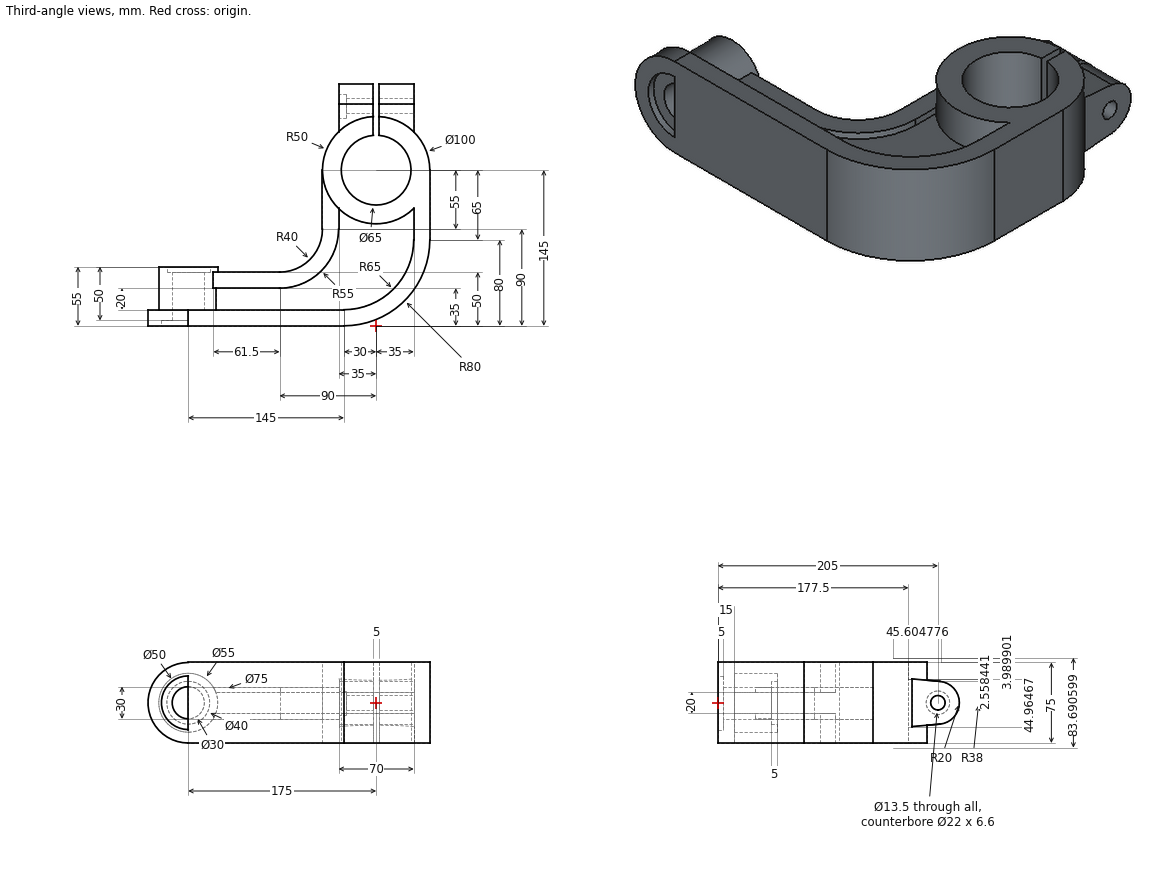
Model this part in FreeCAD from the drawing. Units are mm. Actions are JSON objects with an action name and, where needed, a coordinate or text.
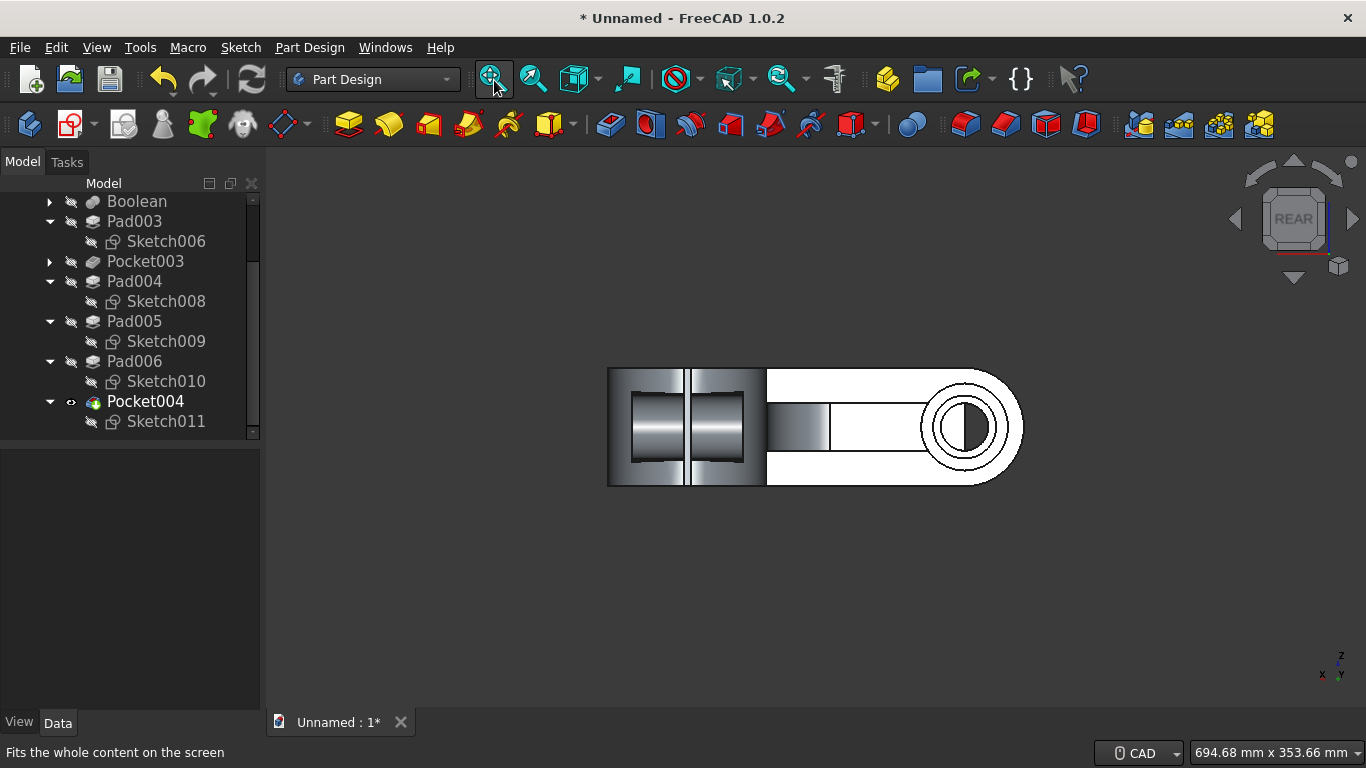
{"action": "key", "text": "6"}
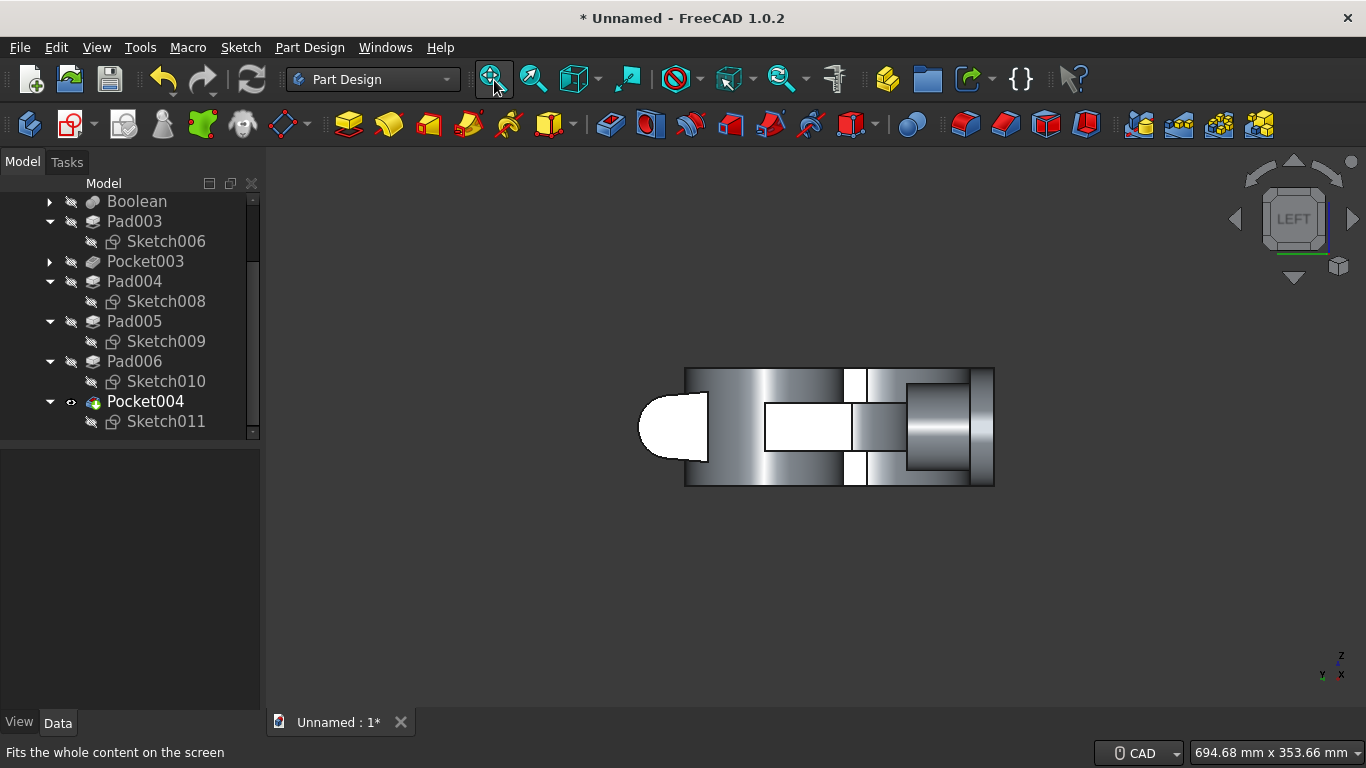
{"action": "key", "text": "v f"}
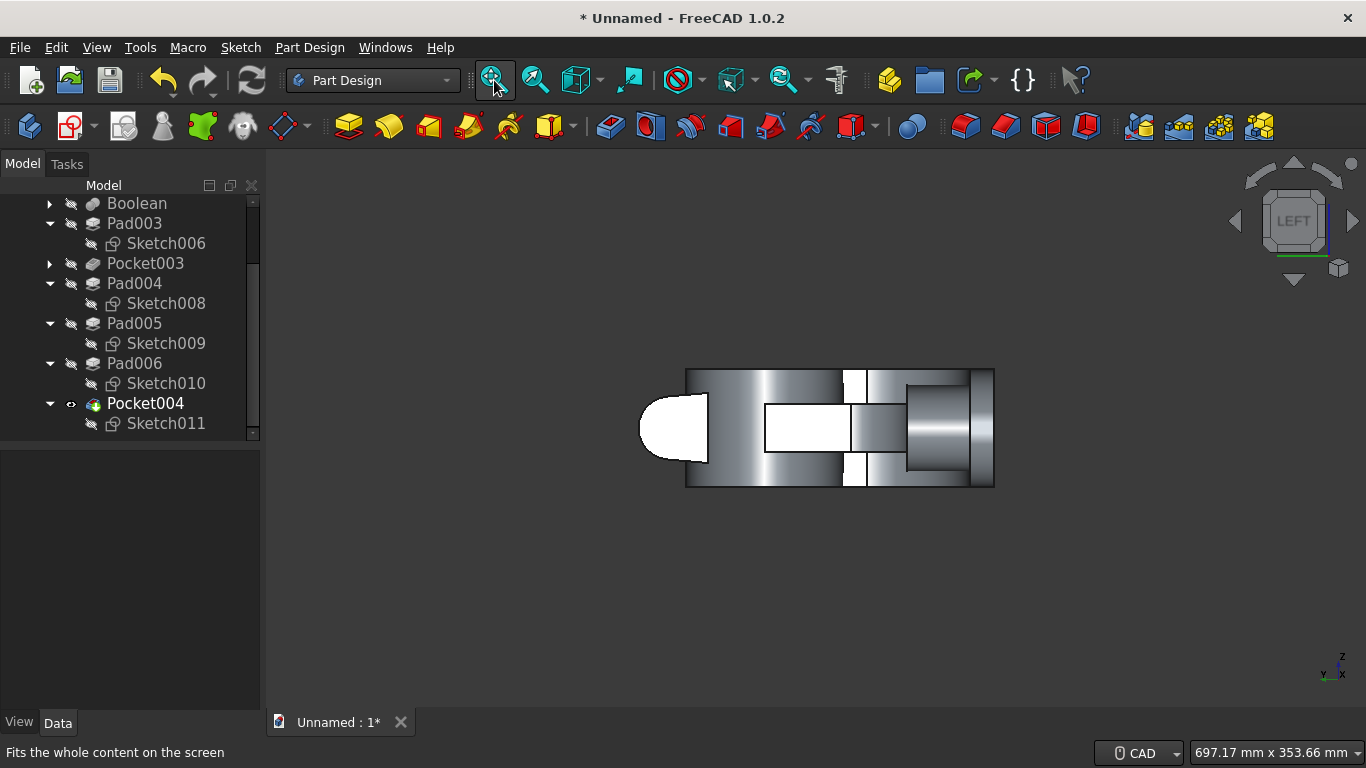
{"action": "left_click", "coordinate": [673, 427]}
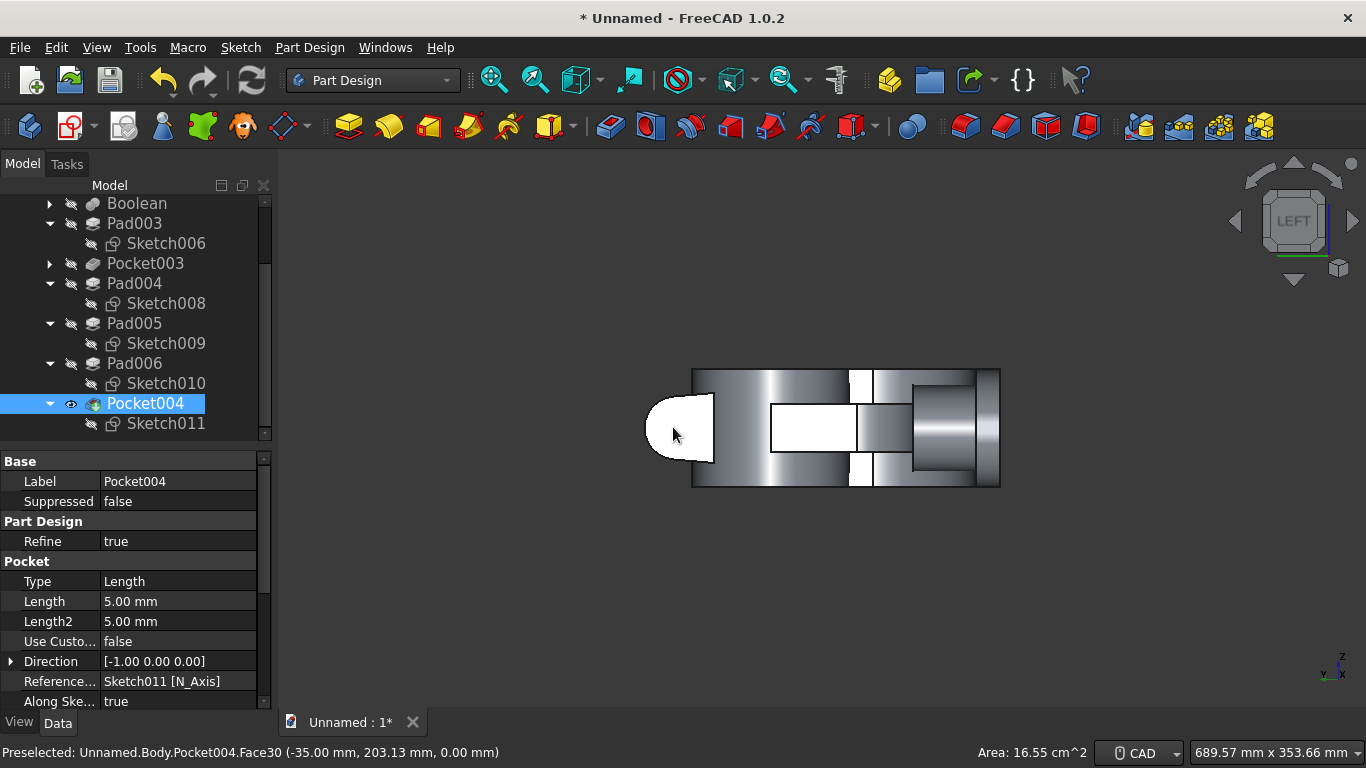
{"action": "left_click", "coordinate": [70, 126]}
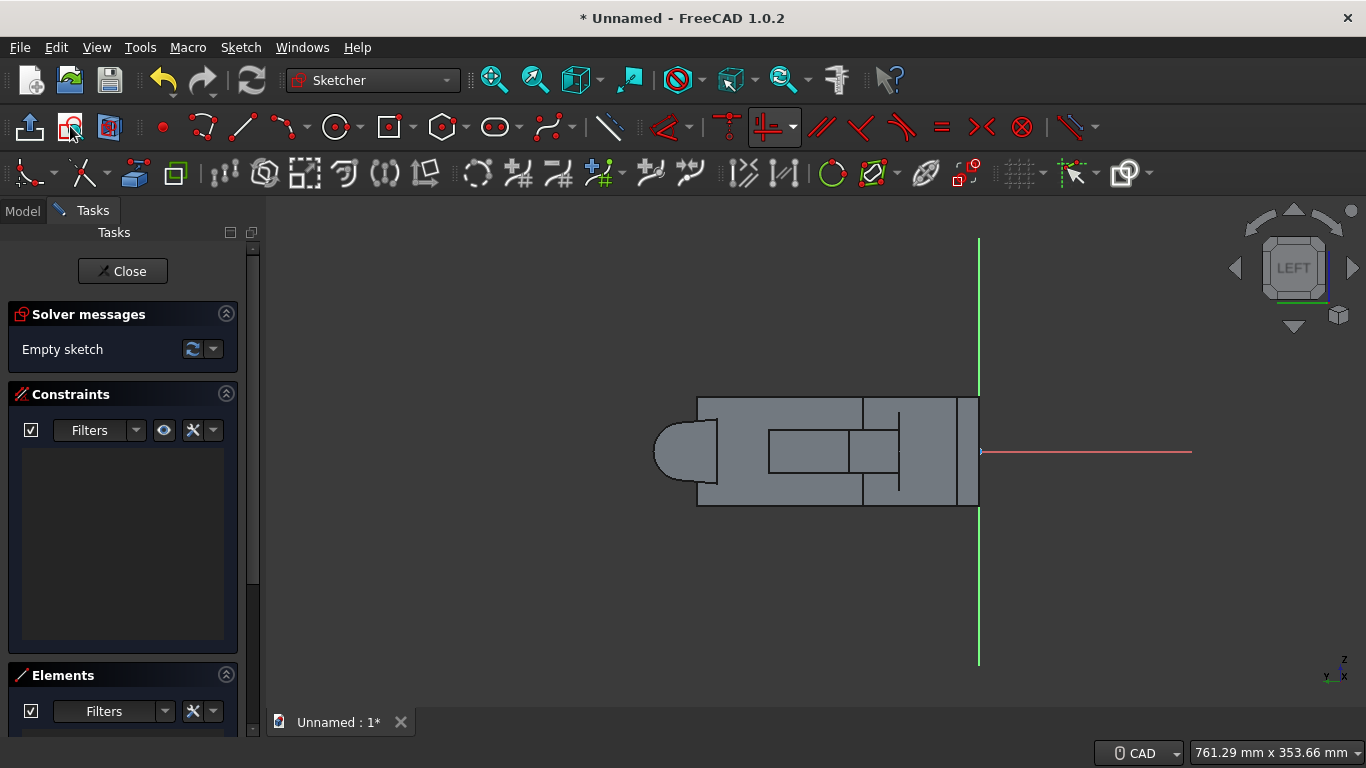
{"action": "key", "text": "q s"}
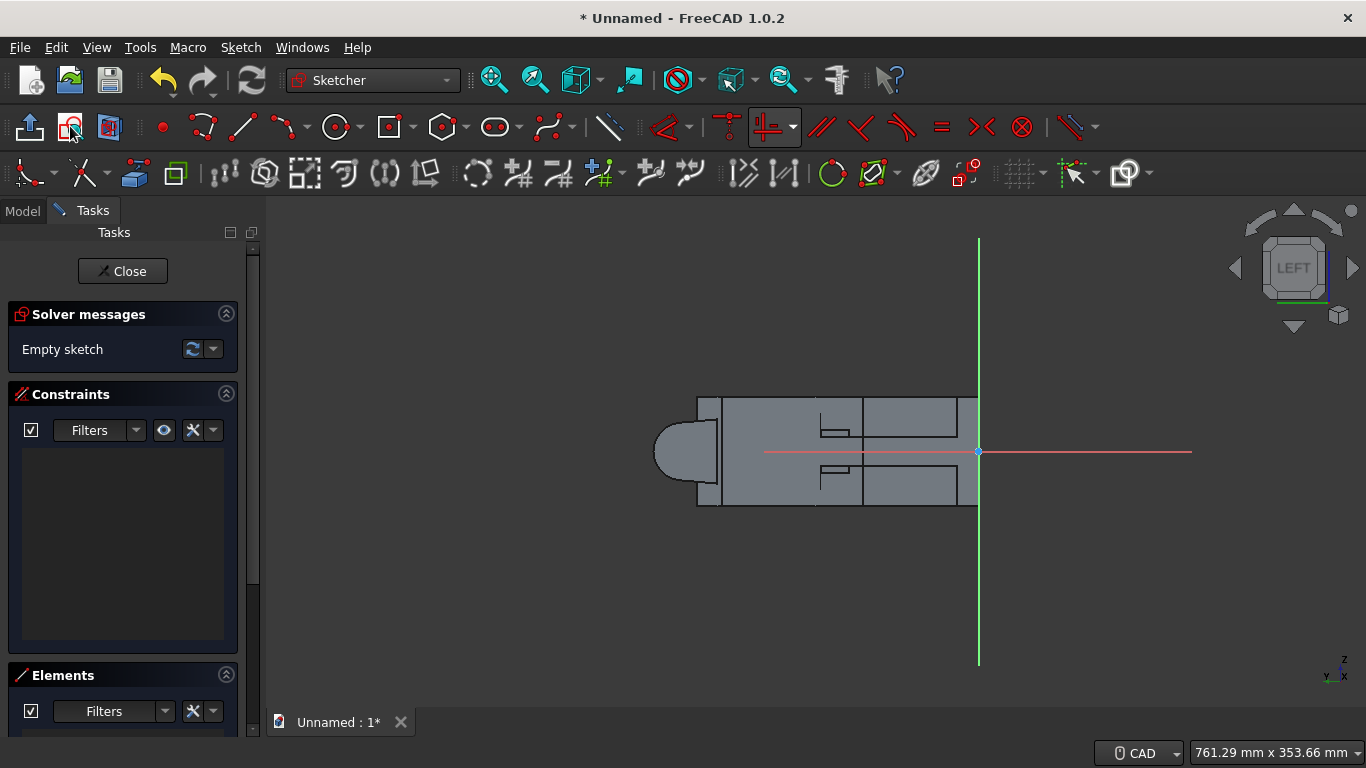
{"action": "scroll", "coordinate": [678, 452], "scroll_direction": "up", "scroll_amount": 14}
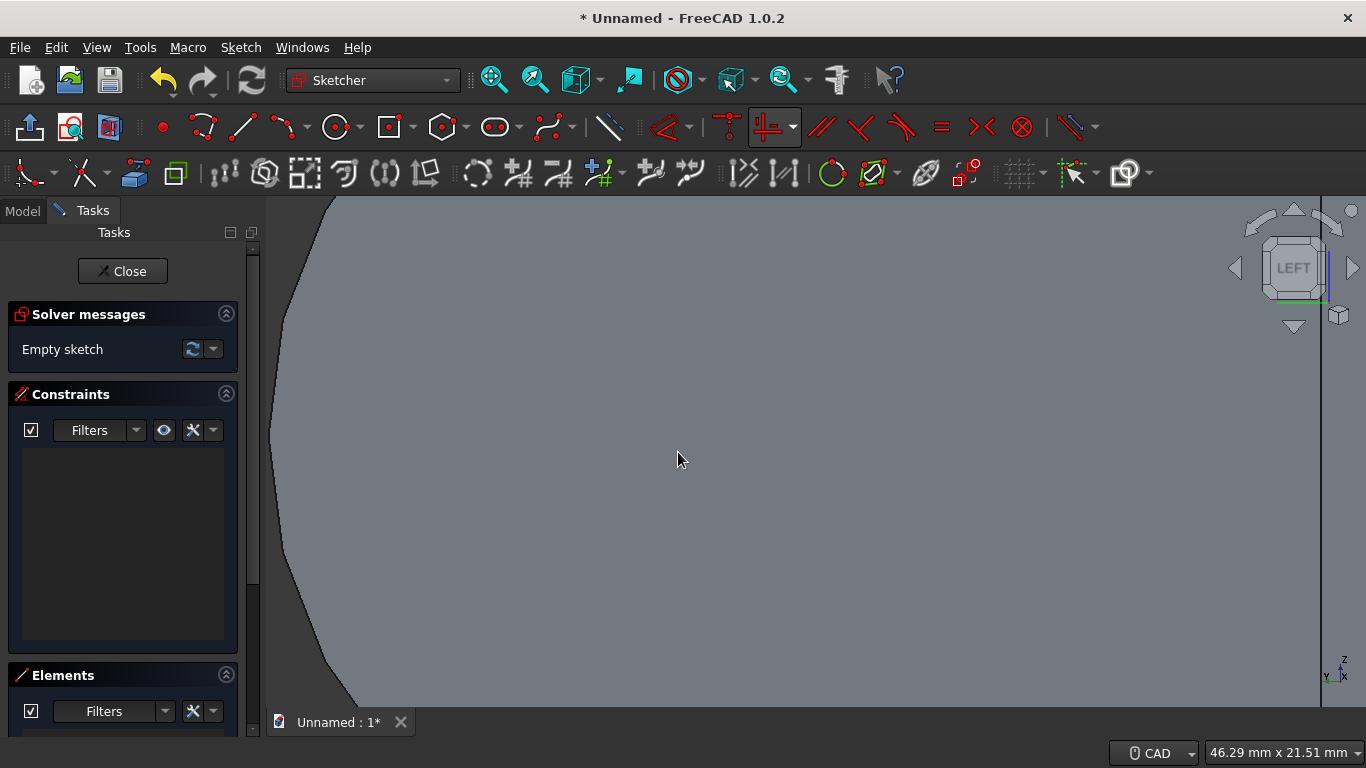
{"action": "key", "text": "g c"}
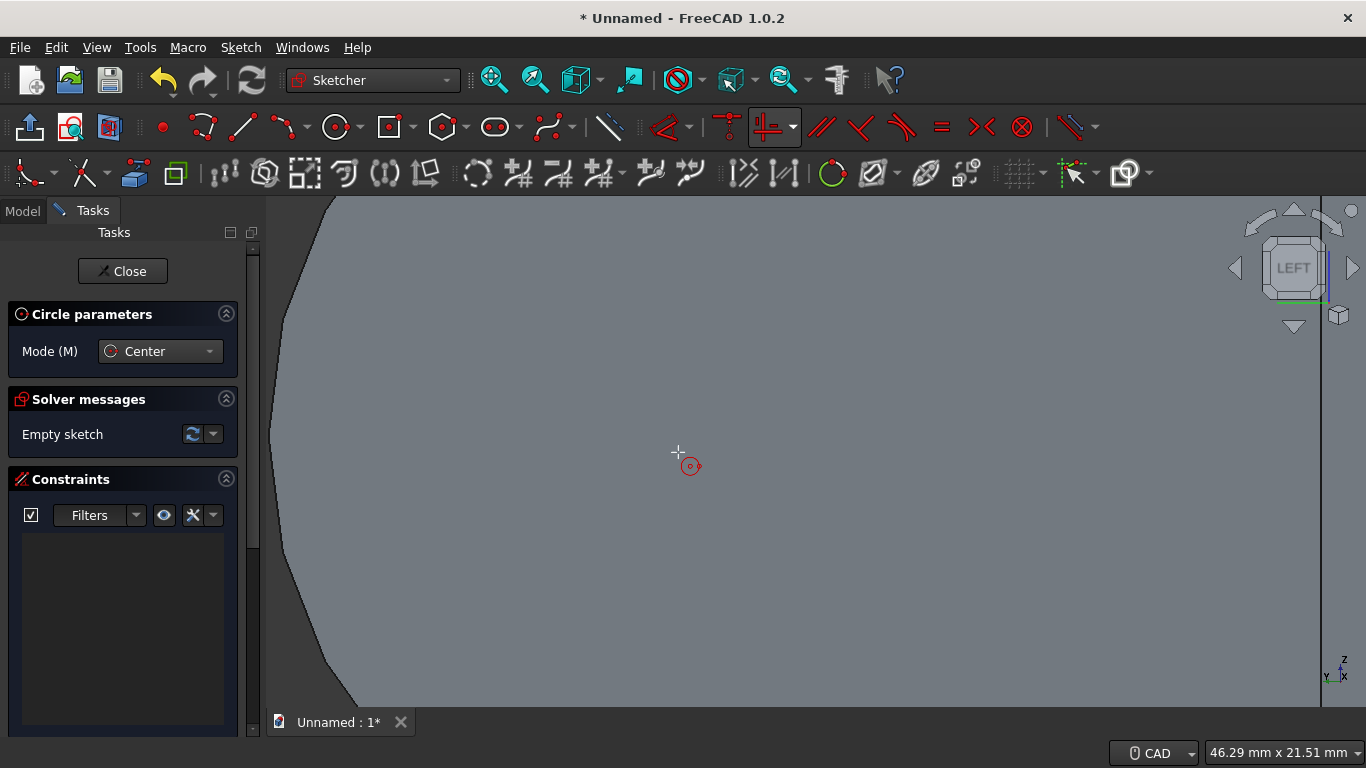
{"action": "left_click", "coordinate": [744, 436]}
{"action": "left_click", "coordinate": [857, 323]}
{"action": "key", "text": "Escape"}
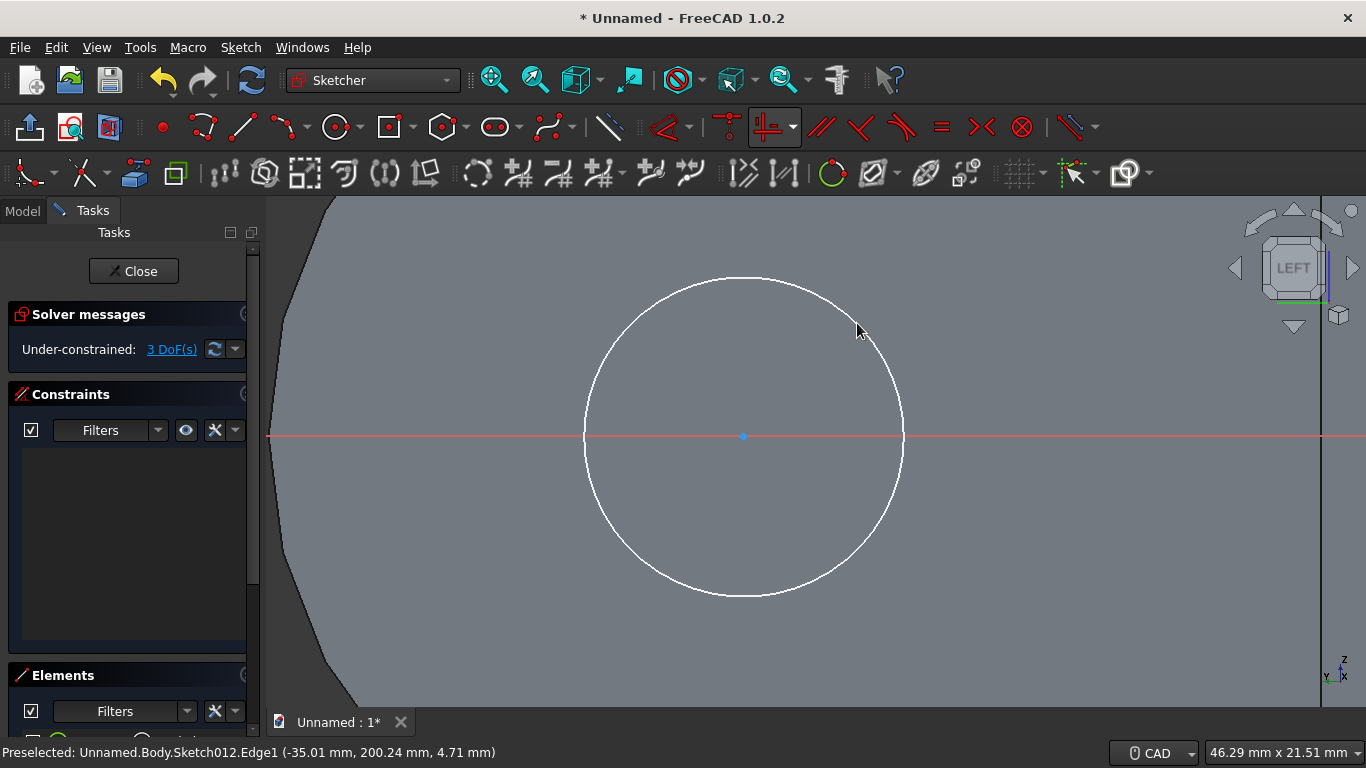
{"action": "left_click", "coordinate": [744, 437]}